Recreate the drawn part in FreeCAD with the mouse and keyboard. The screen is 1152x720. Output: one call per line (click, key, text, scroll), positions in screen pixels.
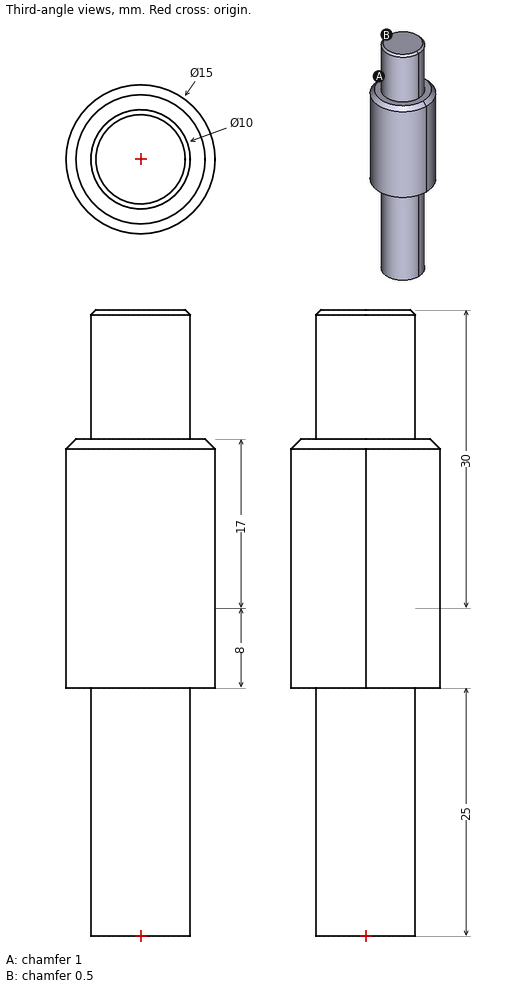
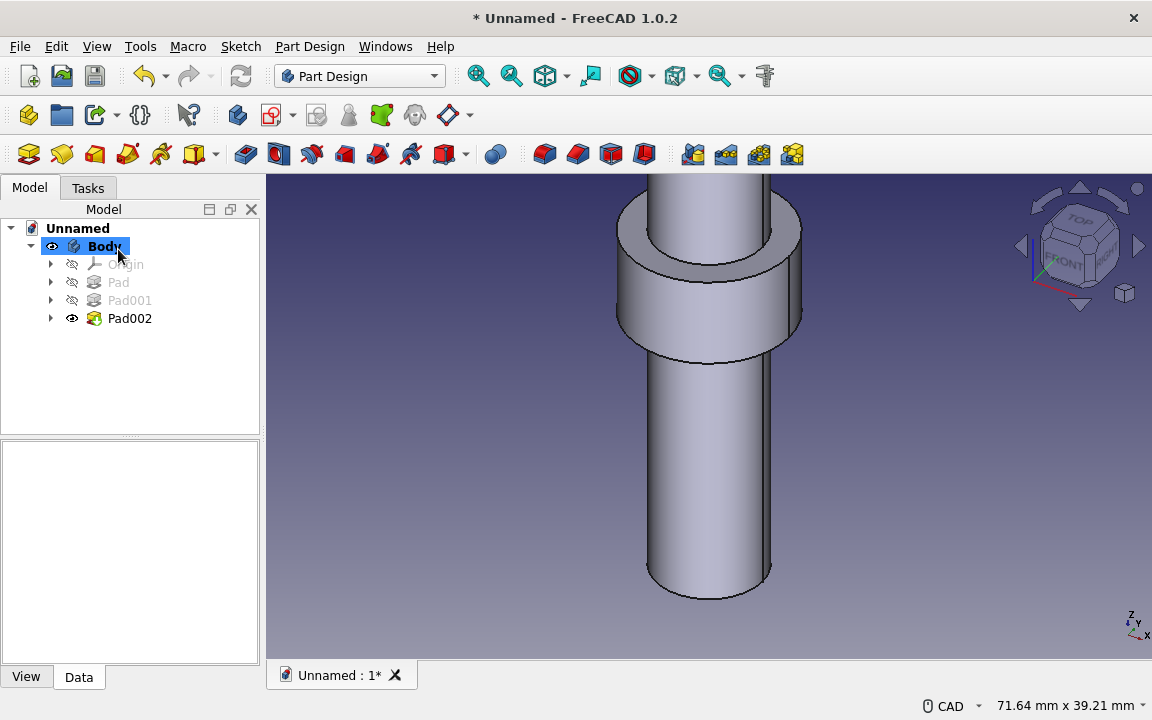
key(v)
key(f)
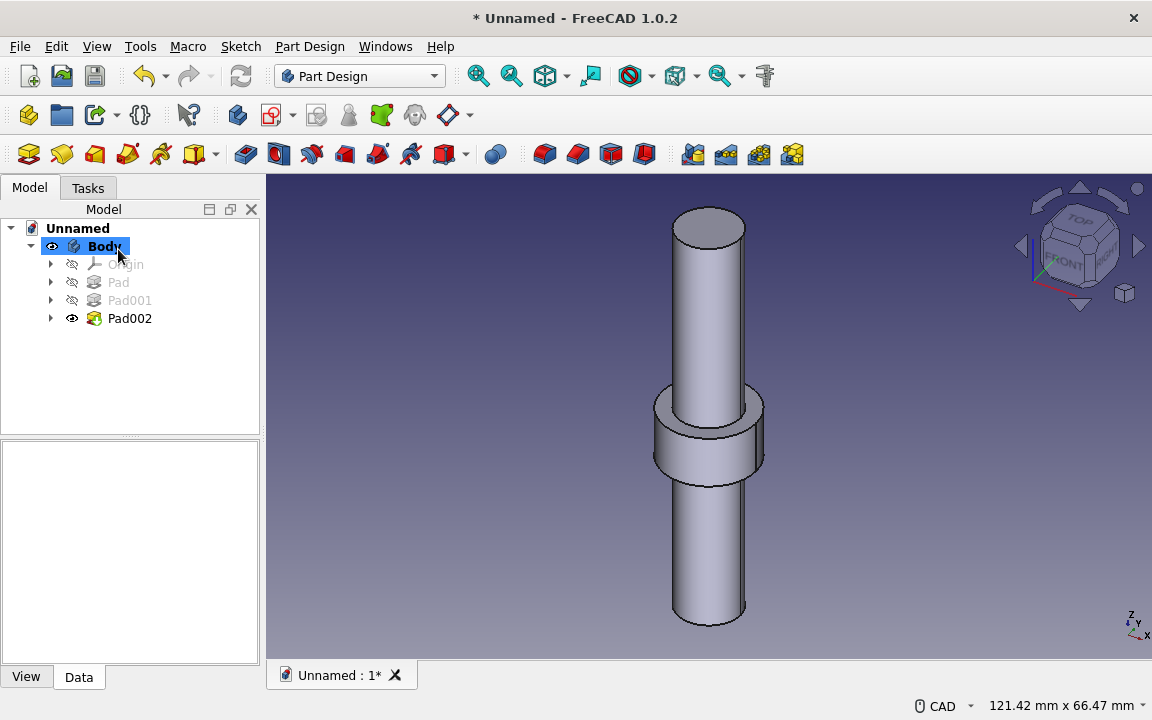
click(666, 413)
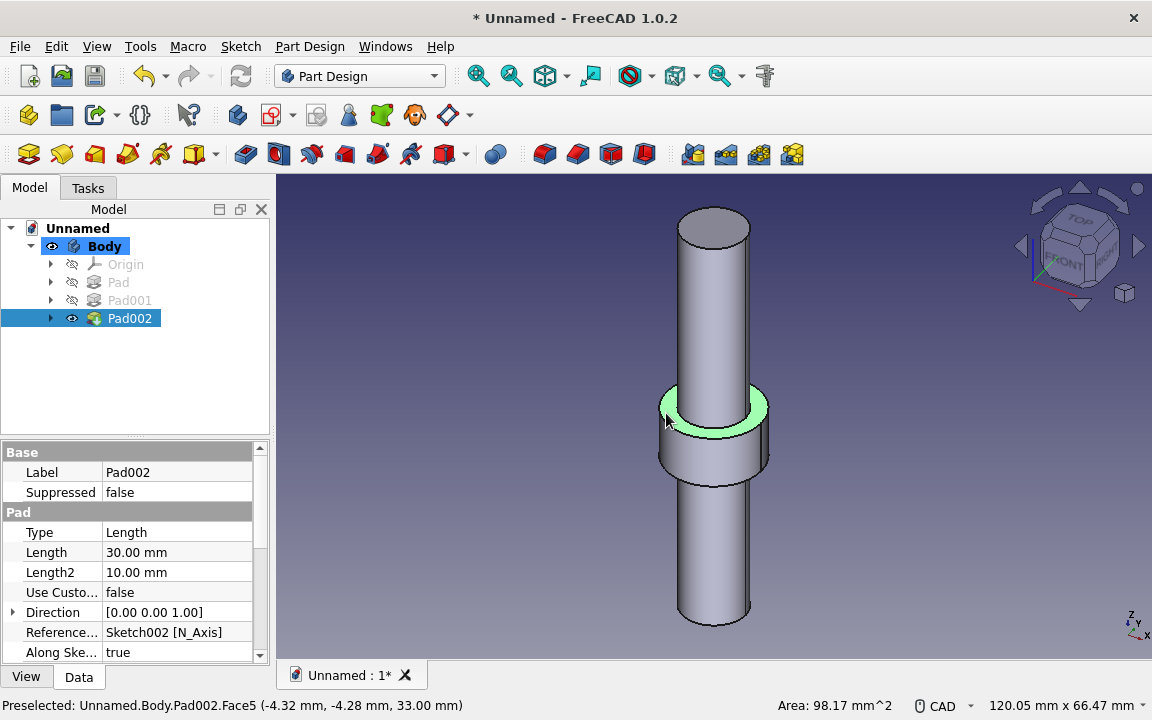
click(270, 116)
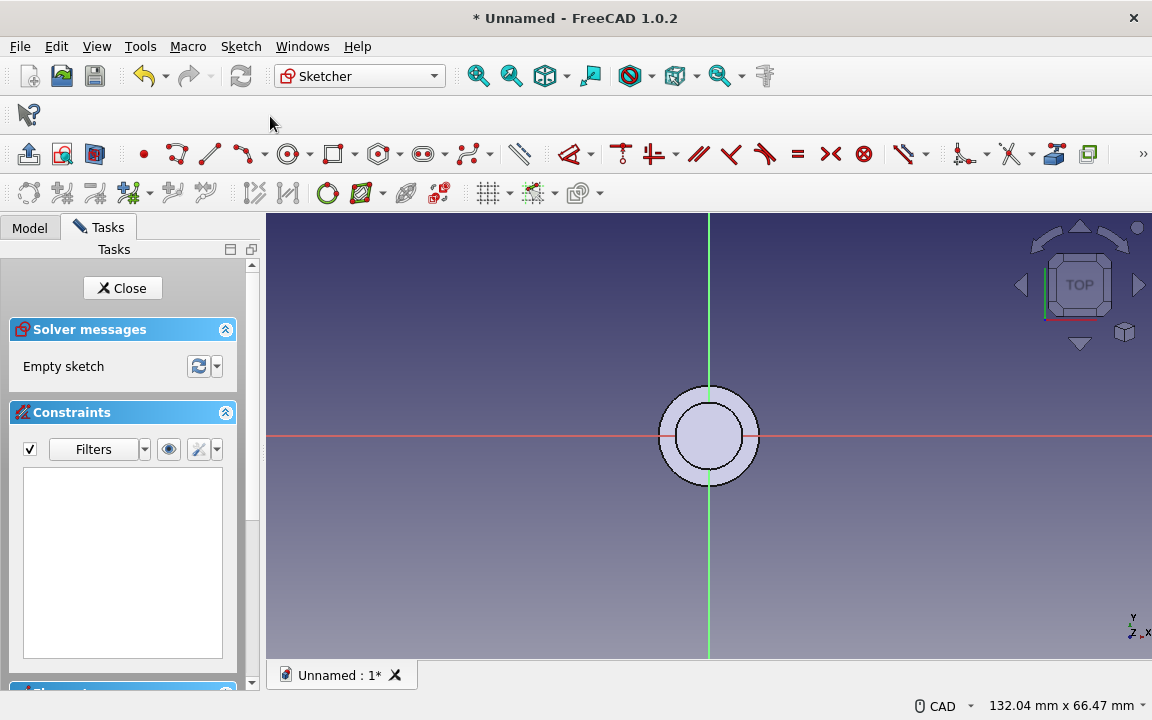
key(q)
key(s)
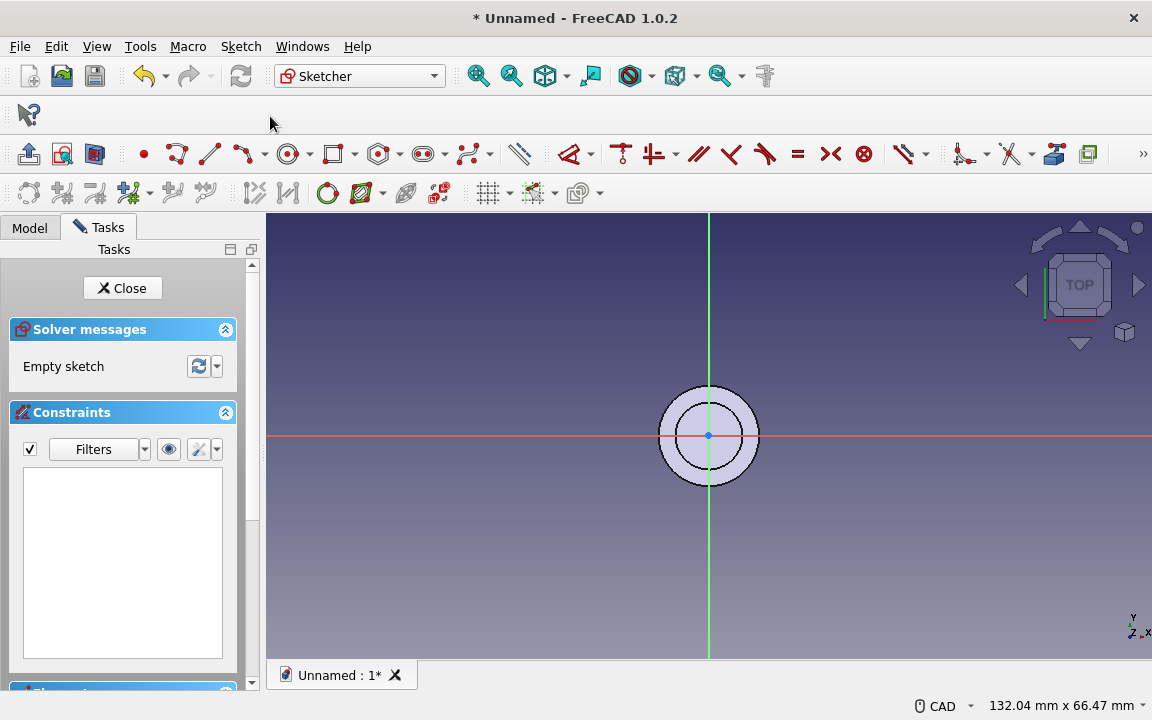
scroll(749, 436, up, 5)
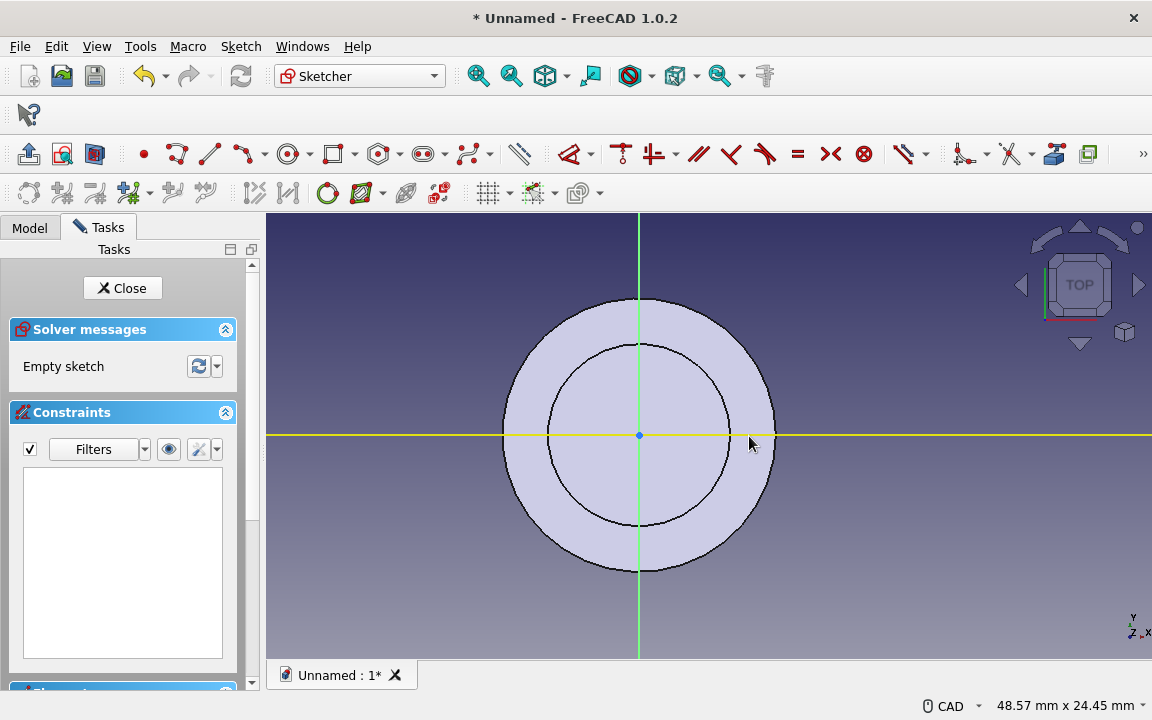
click(288, 154)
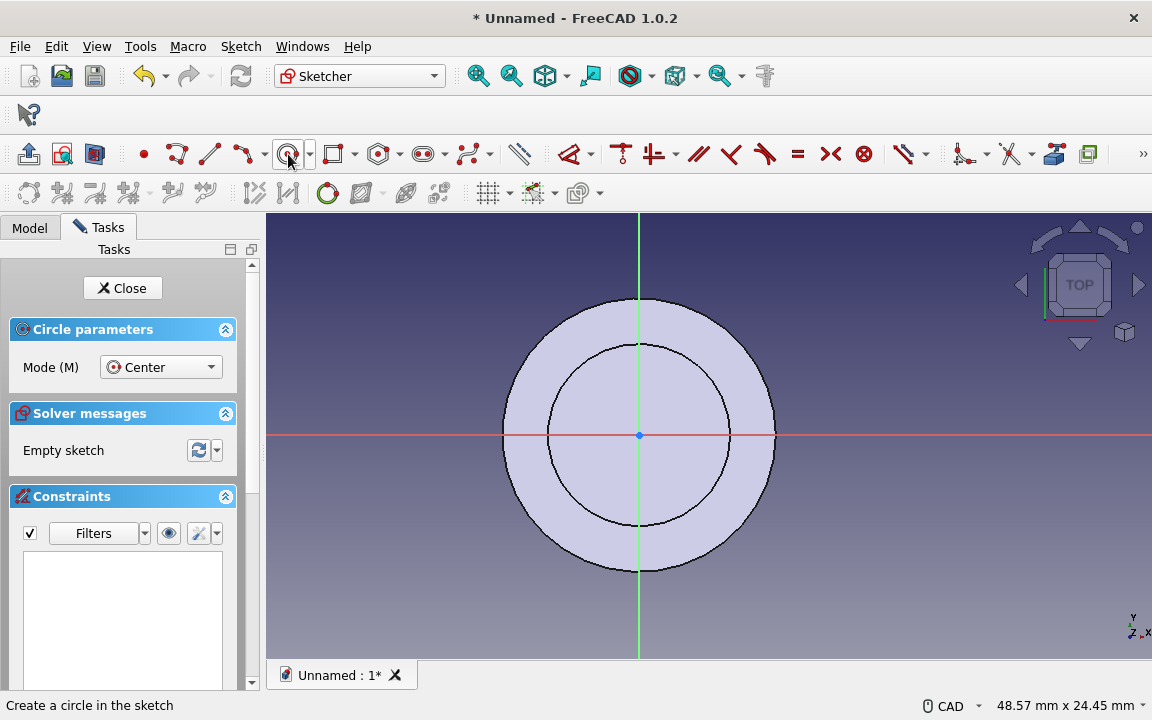
click(639, 435)
click(736, 338)
key(Escape)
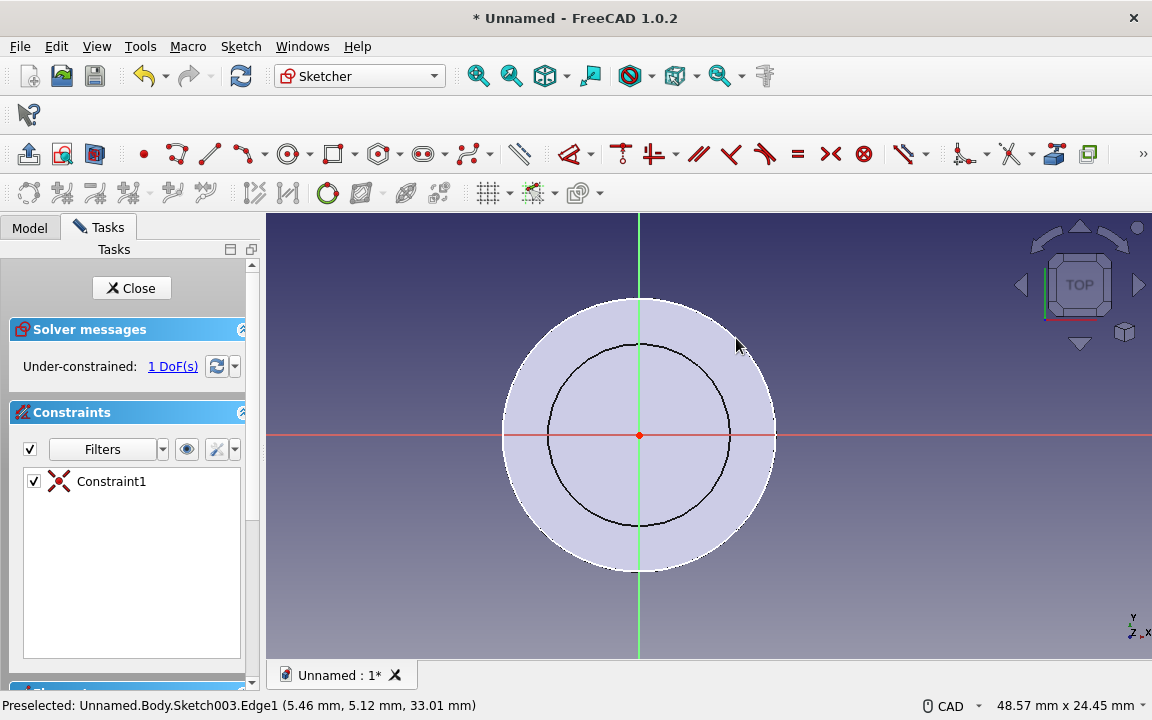
key(d)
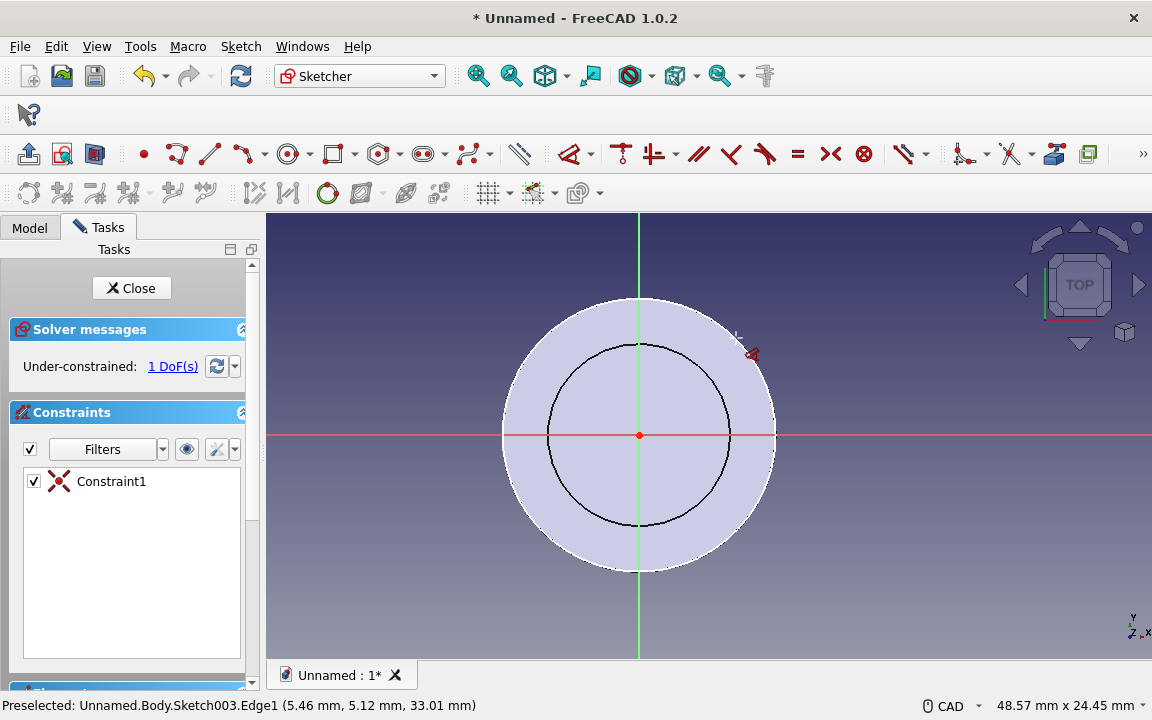
click(735, 338)
click(757, 315)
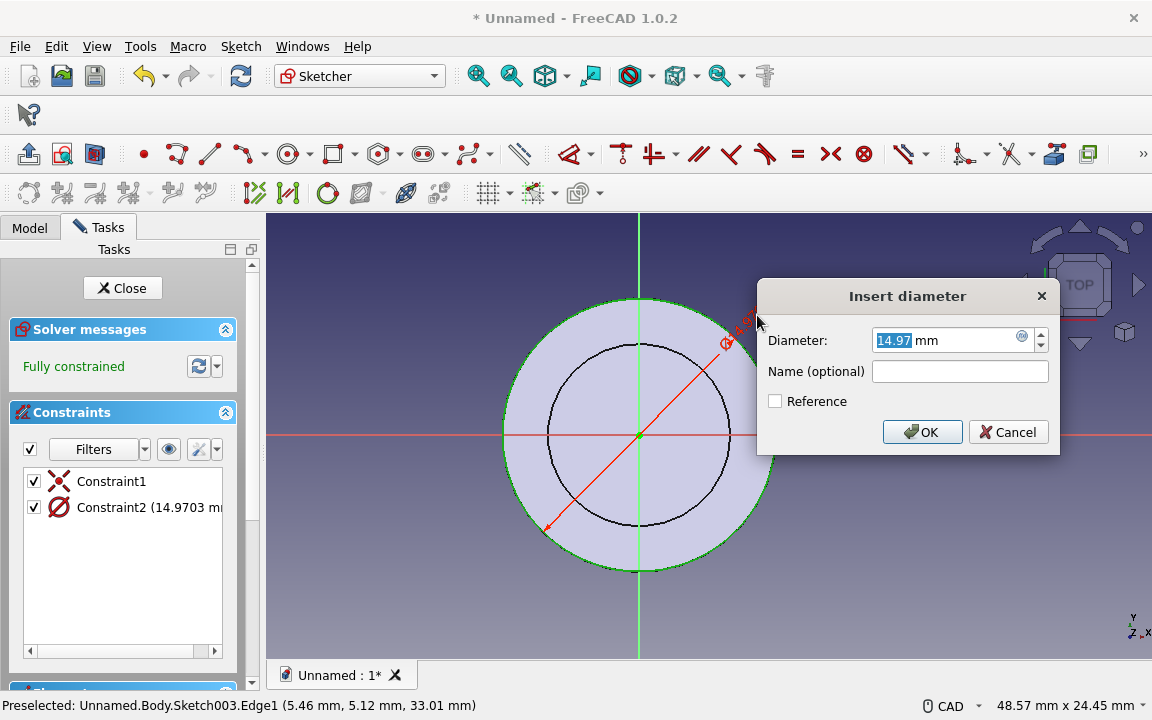
text(15)
key(Return)
key(Escape)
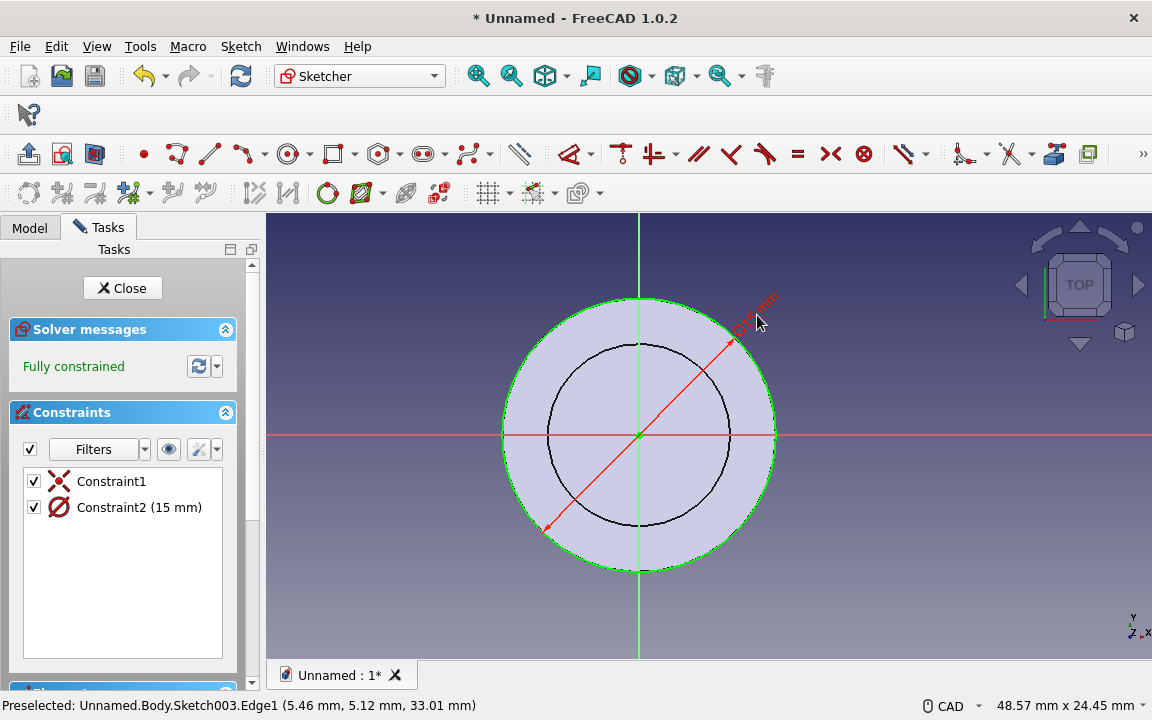
click(123, 288)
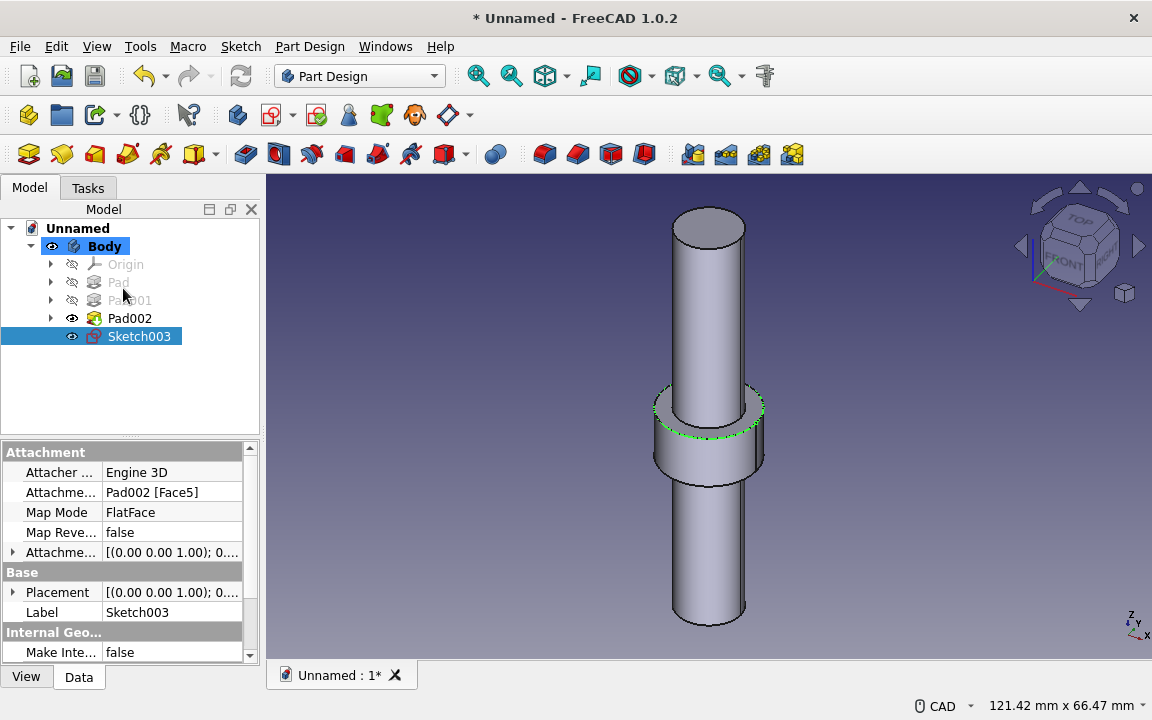
click(29, 154)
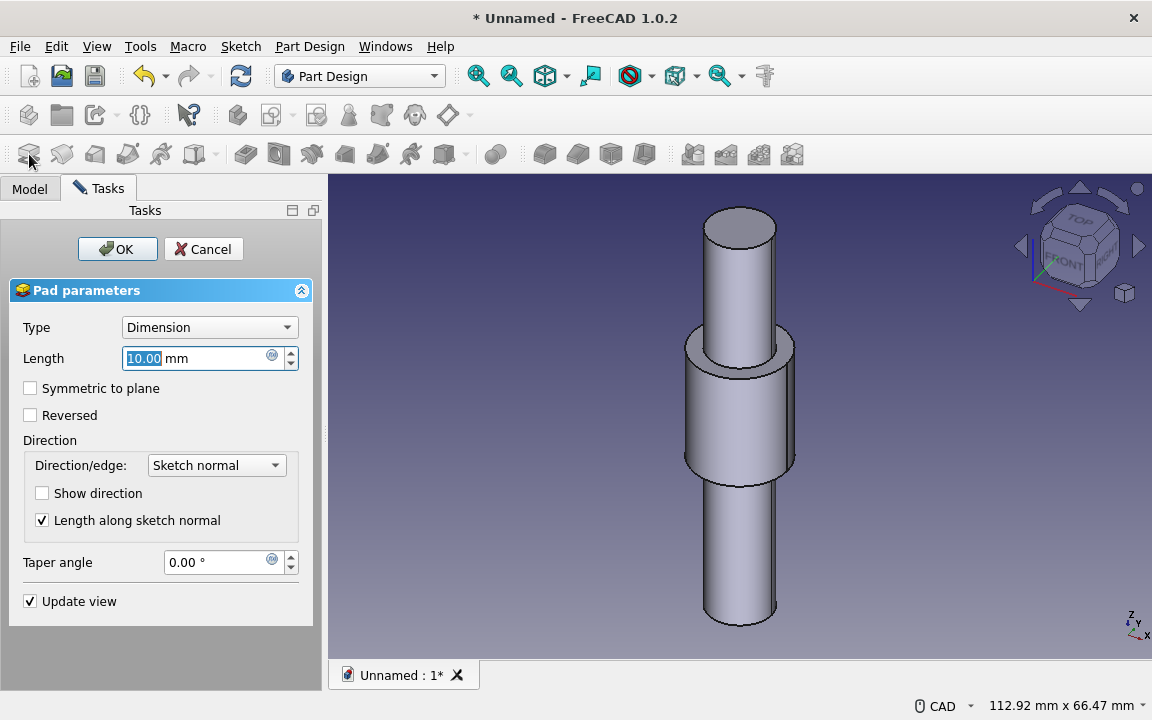
text(17)
key(Tab)